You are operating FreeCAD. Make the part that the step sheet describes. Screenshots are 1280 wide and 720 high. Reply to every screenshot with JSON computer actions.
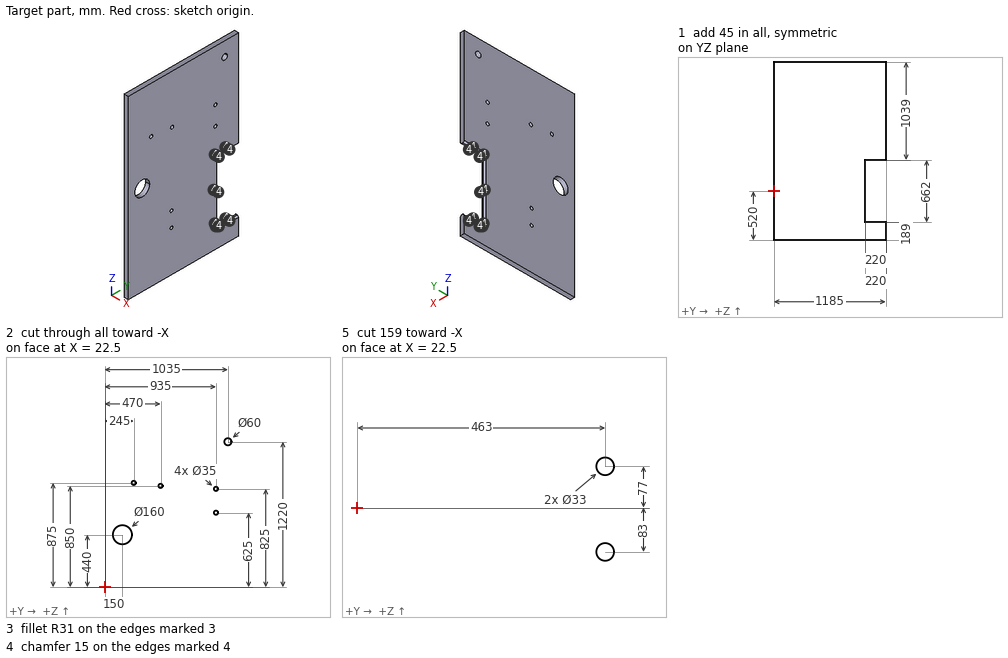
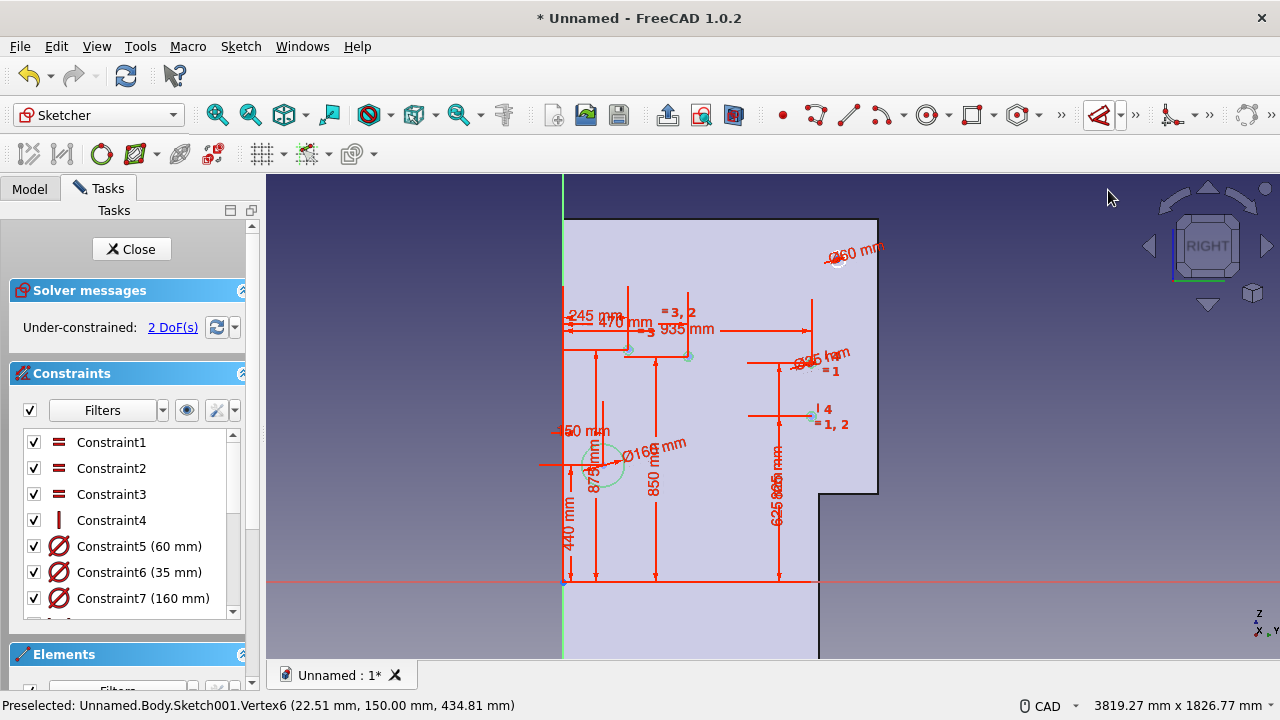
{"action": "left_click", "coordinate": [838, 259]}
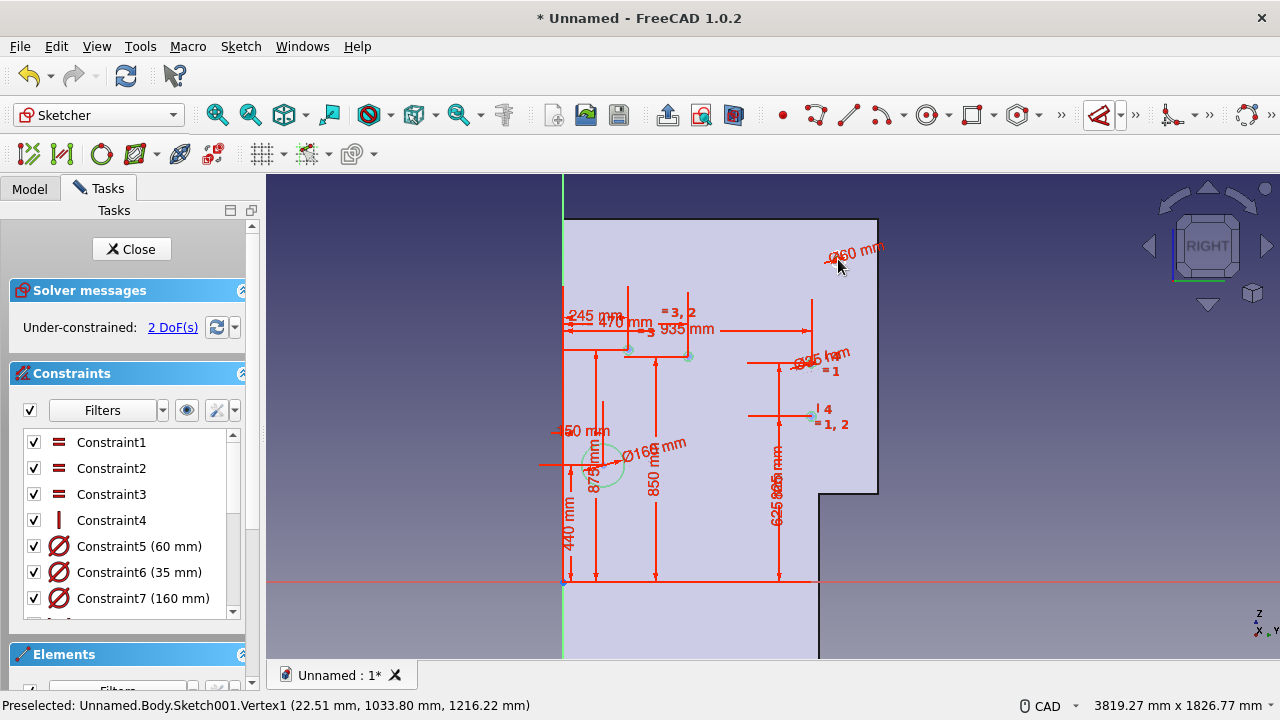
{"action": "key", "text": "l"}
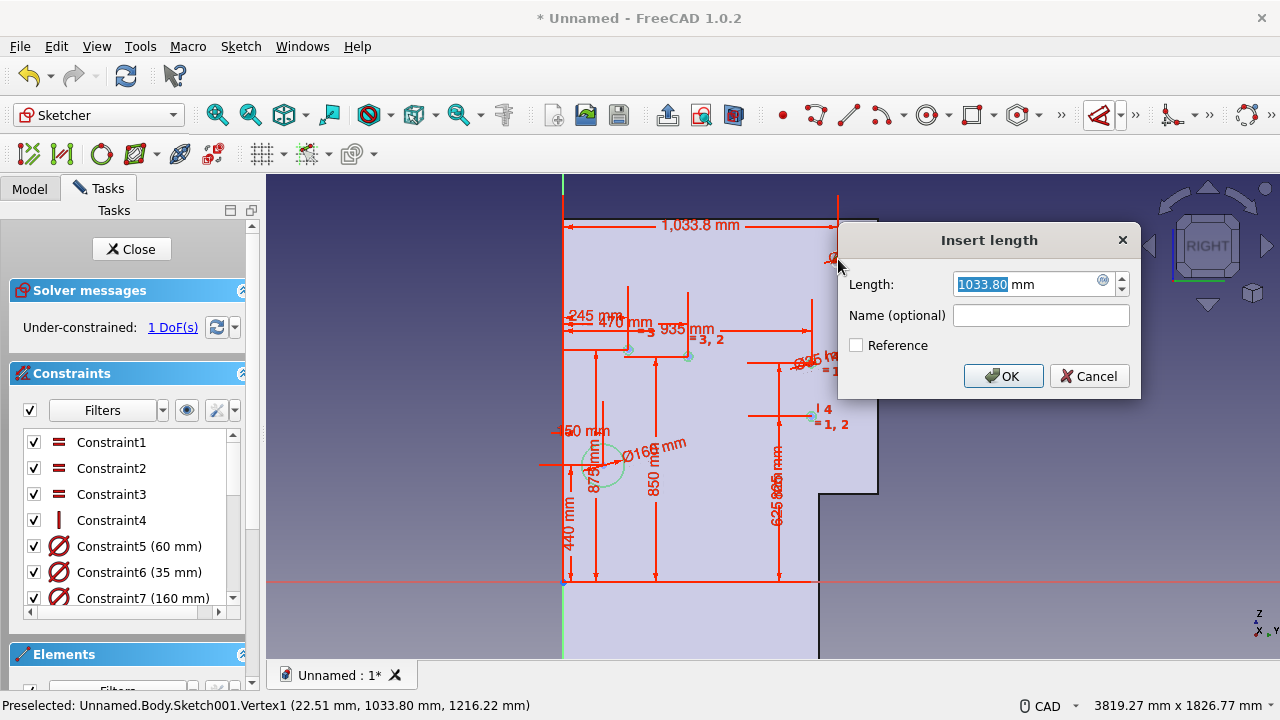
{"action": "type", "text": "1035"}
{"action": "key", "text": "Return"}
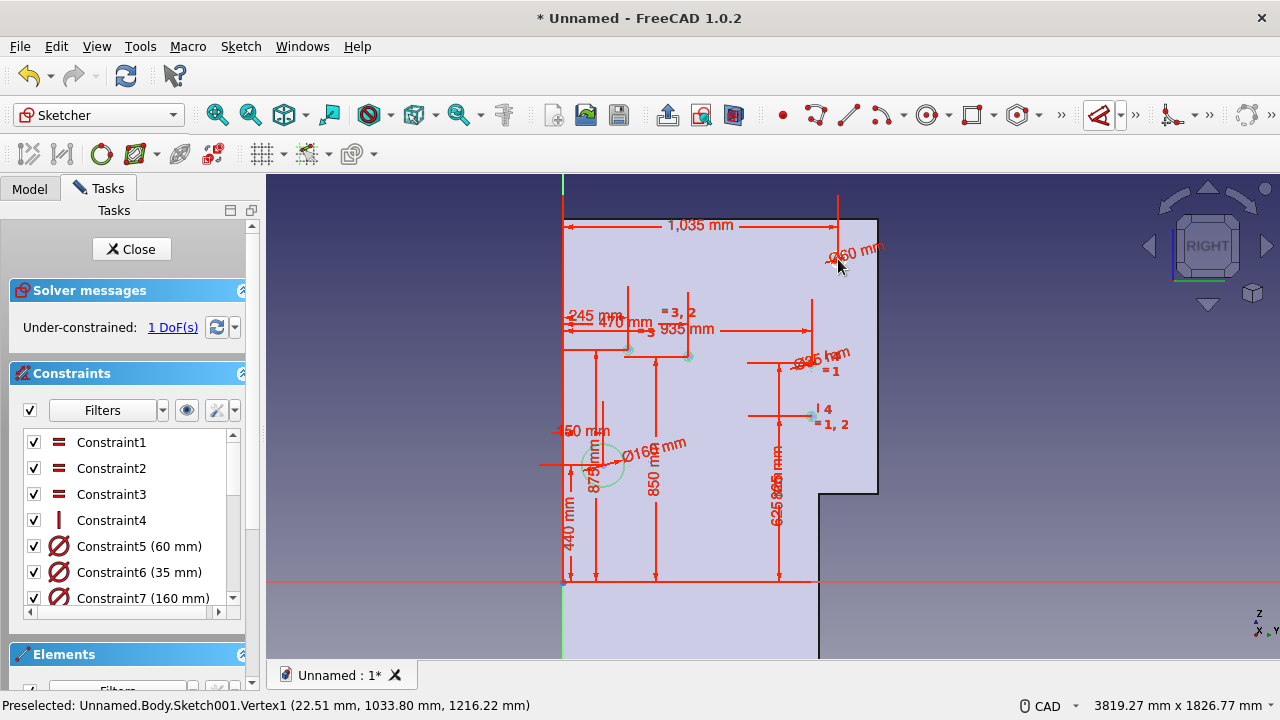
{"action": "left_click", "coordinate": [838, 259]}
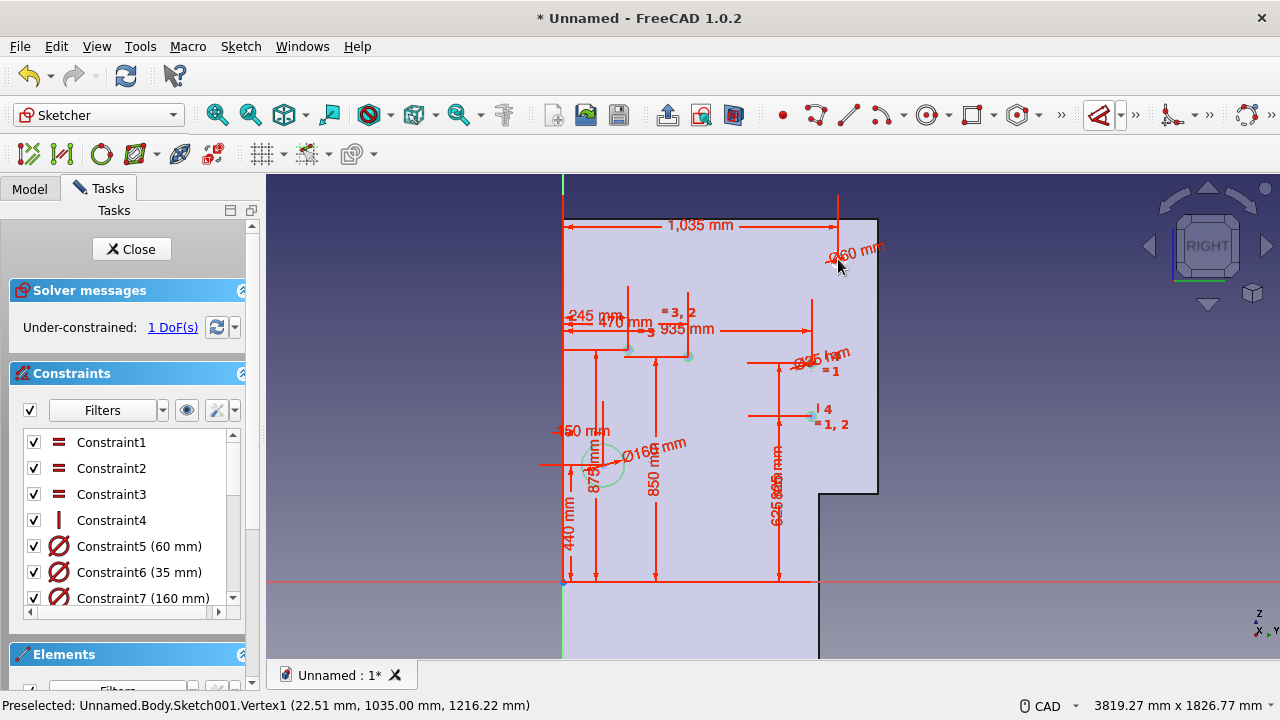
{"action": "left_click", "coordinate": [1120, 116]}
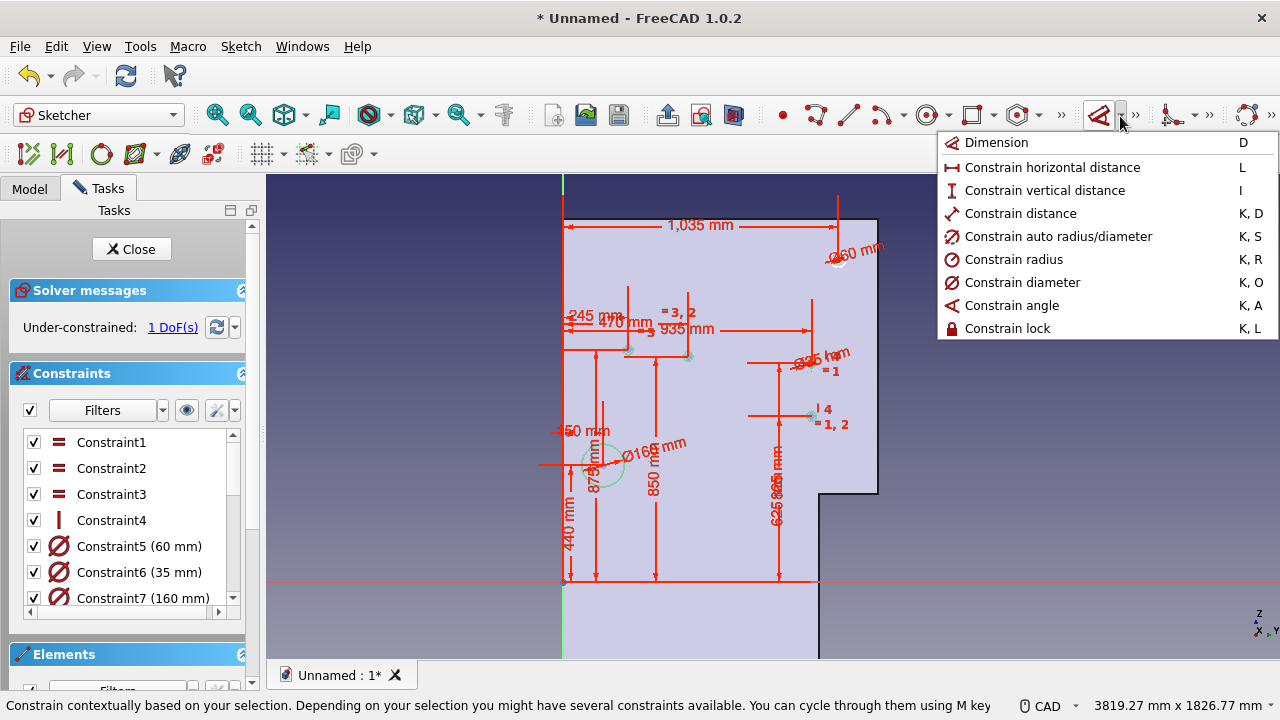
{"action": "left_click", "coordinate": [1108, 190]}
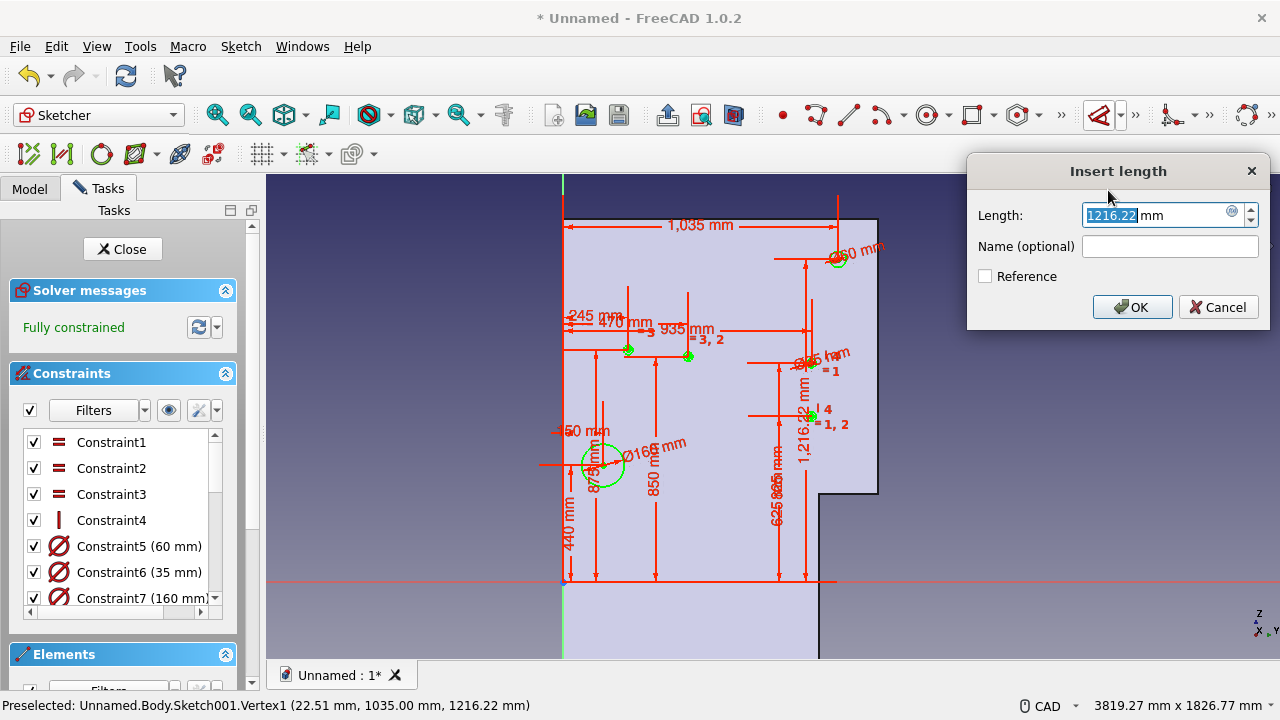
{"action": "type", "text": "1220"}
{"action": "key", "text": "Return"}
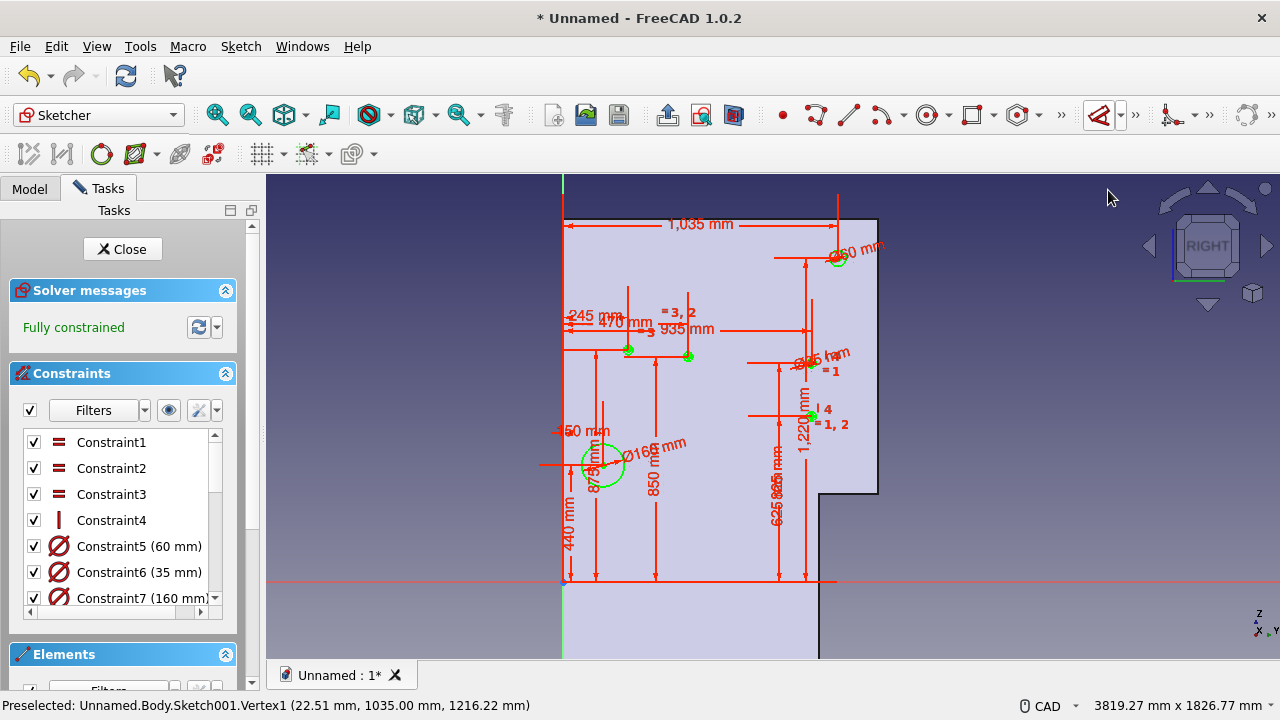
{"action": "left_click", "coordinate": [123, 249]}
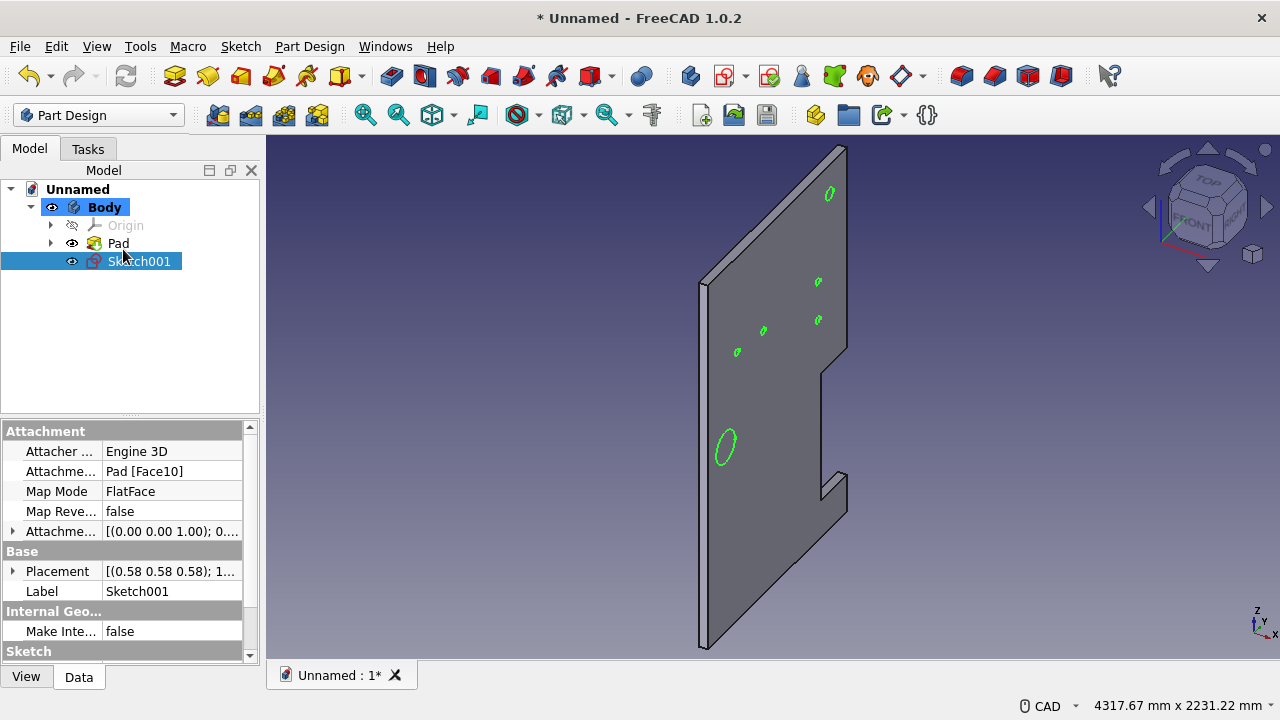
{"action": "left_click", "coordinate": [392, 76]}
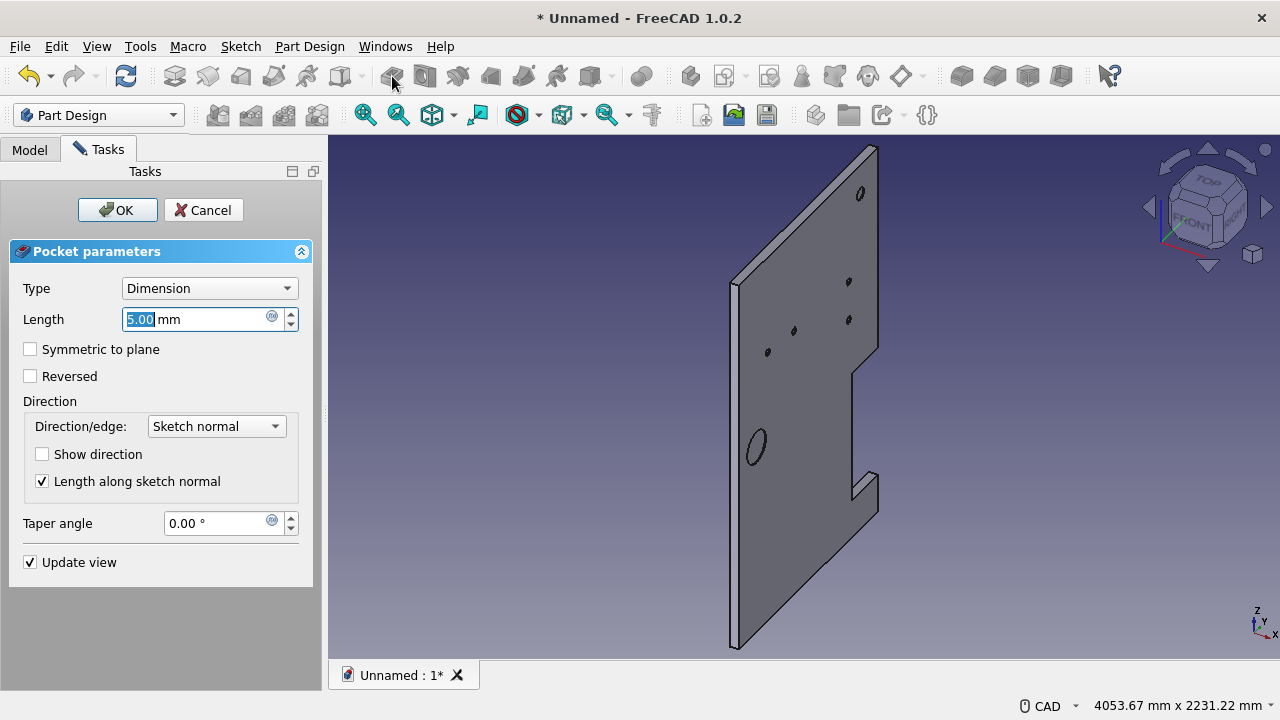
{"action": "left_click", "coordinate": [210, 288]}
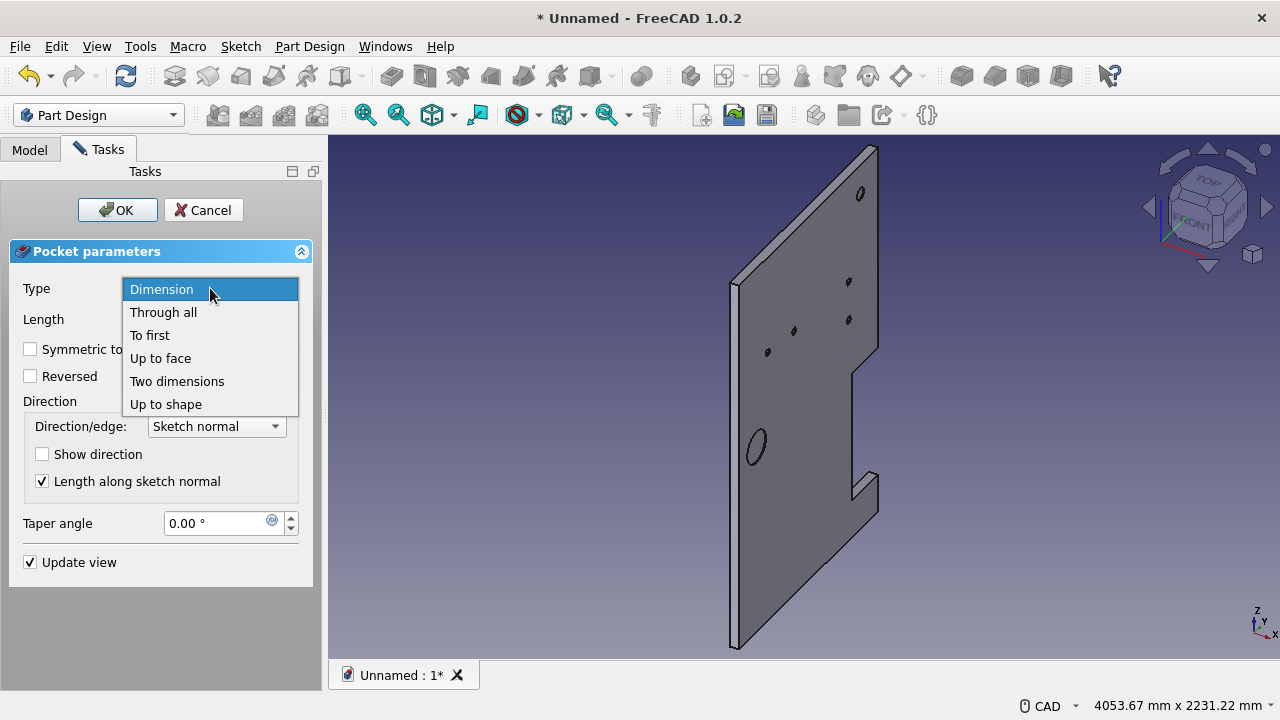
{"action": "left_click", "coordinate": [208, 312]}